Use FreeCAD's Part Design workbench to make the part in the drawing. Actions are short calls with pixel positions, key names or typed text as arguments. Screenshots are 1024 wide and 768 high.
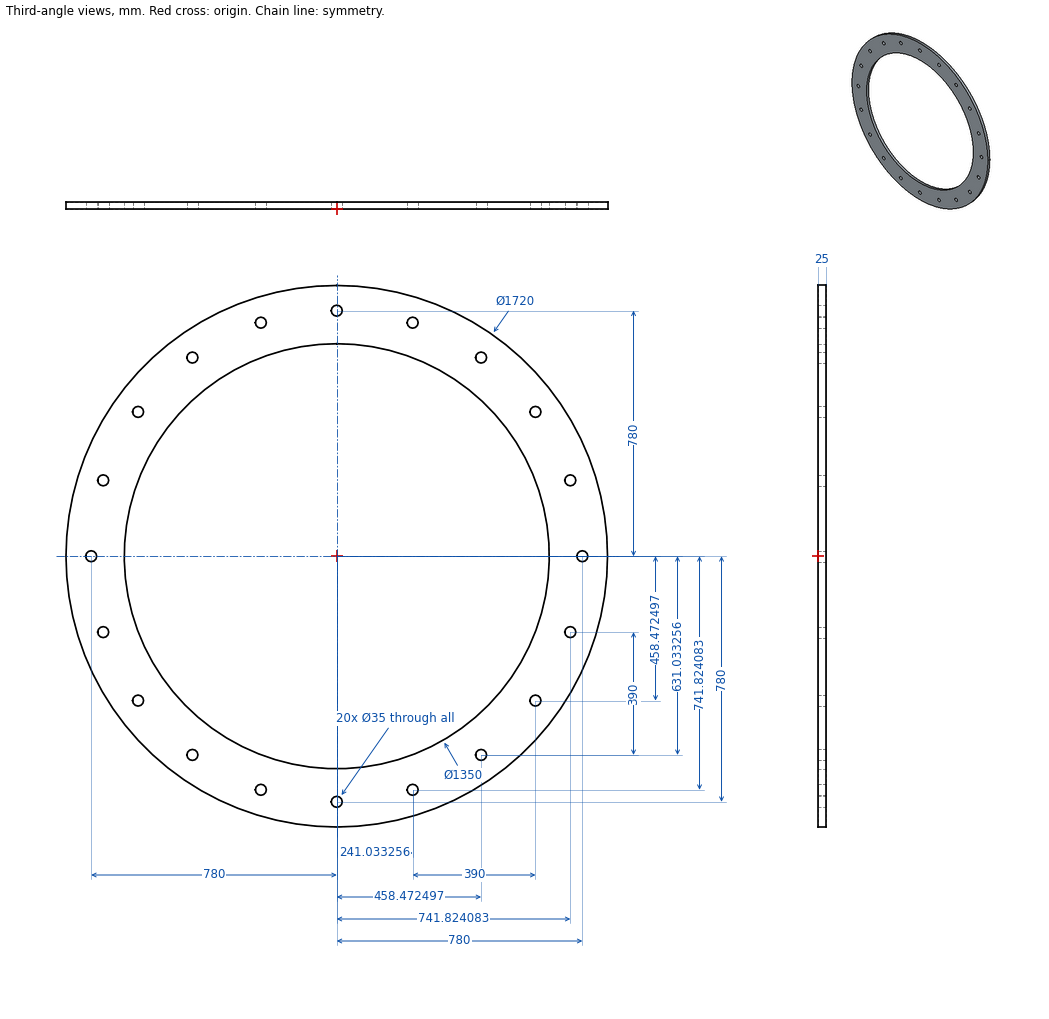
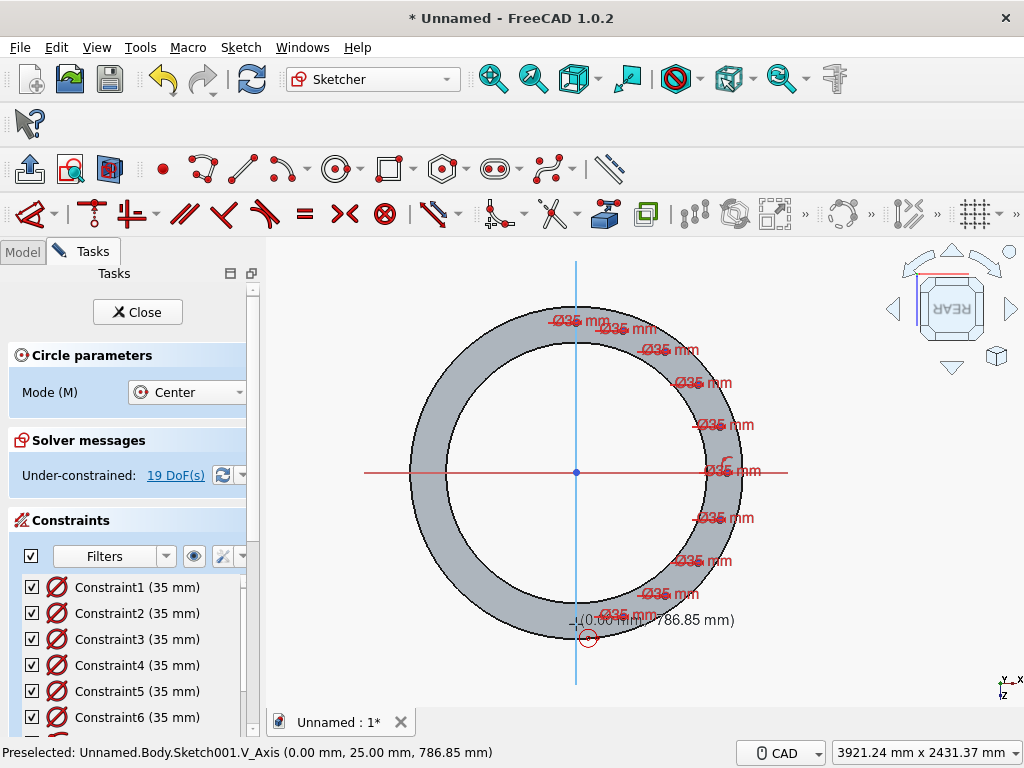
scroll(580, 623, up, 9)
move(576, 616)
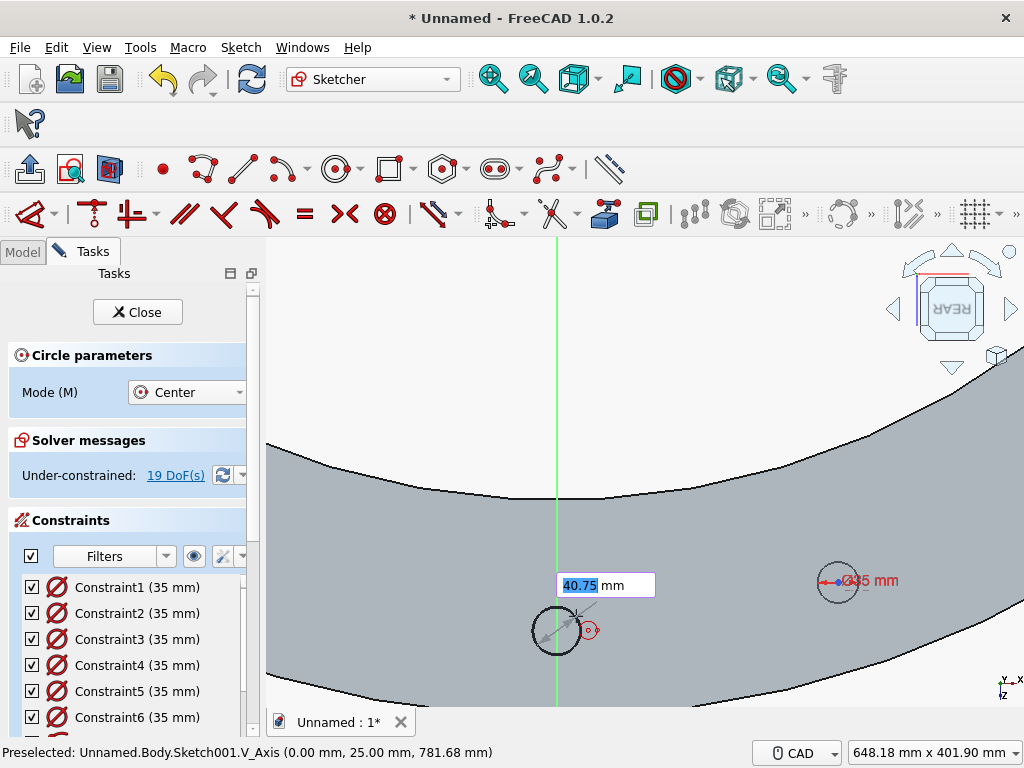
text(35)
key(Return)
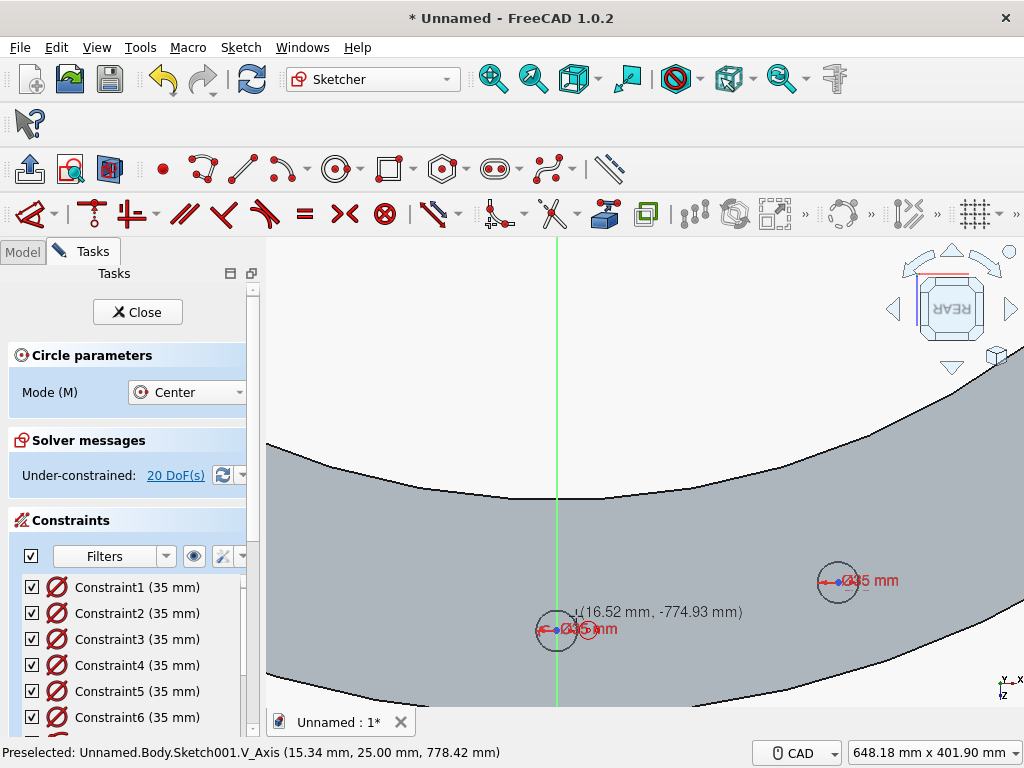
scroll(580, 623, down, 9)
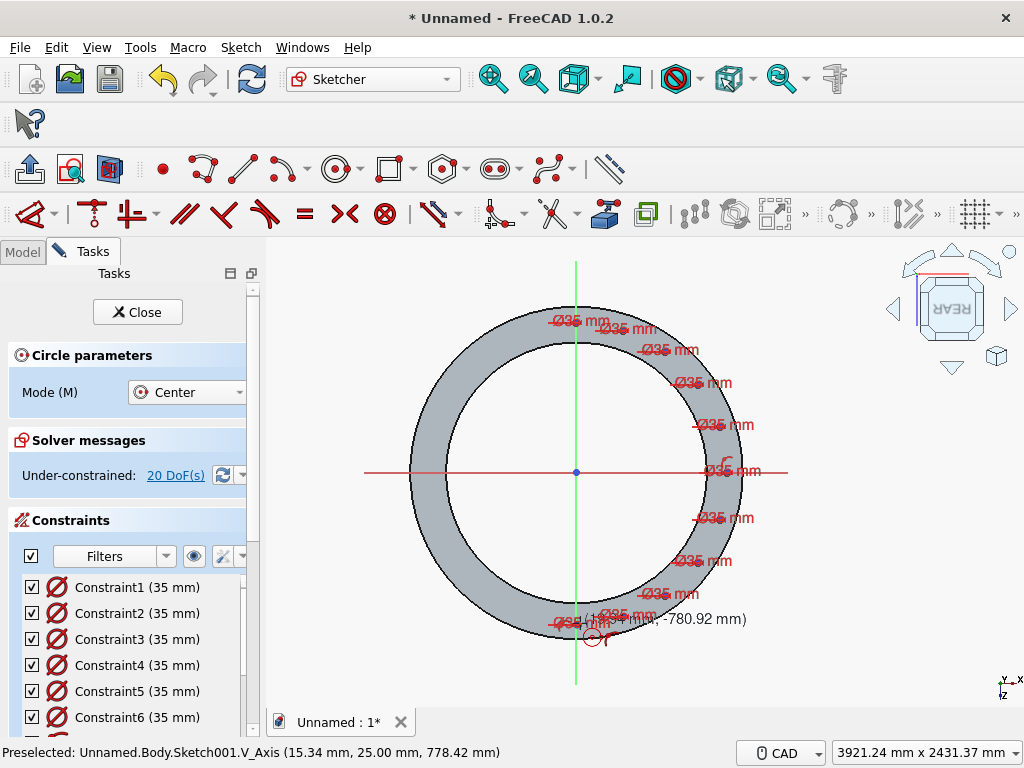
scroll(530, 616, up, 10)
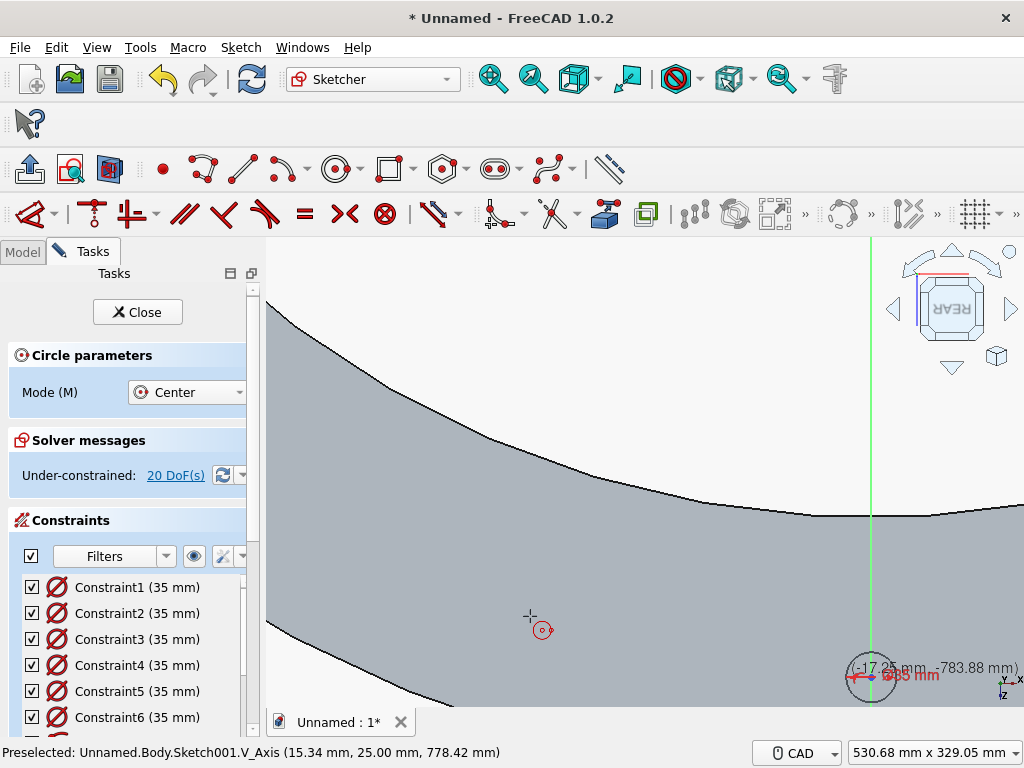
scroll(530, 616, down, 10)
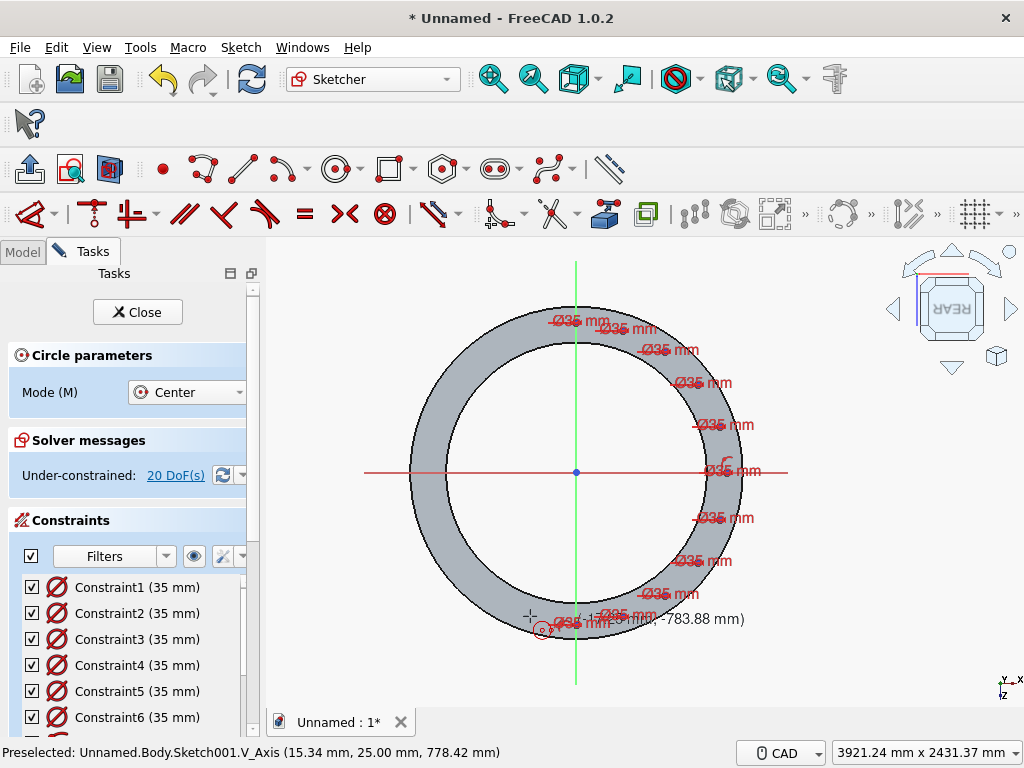
click(530, 616)
move(532, 614)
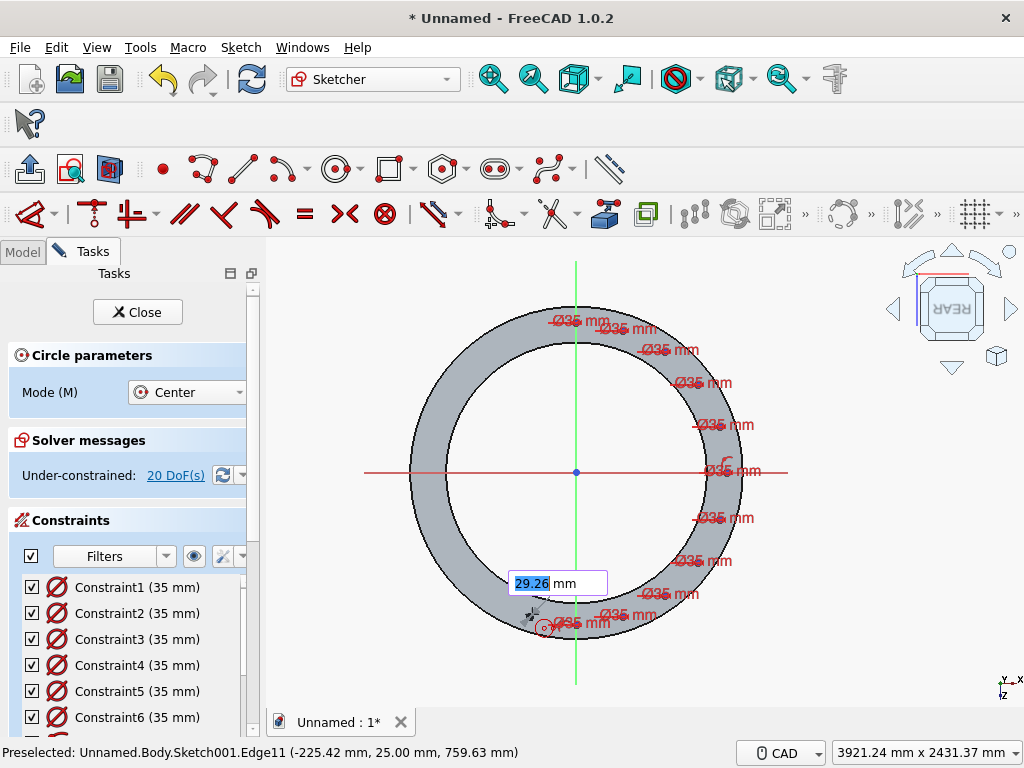
text(35)
key(Return)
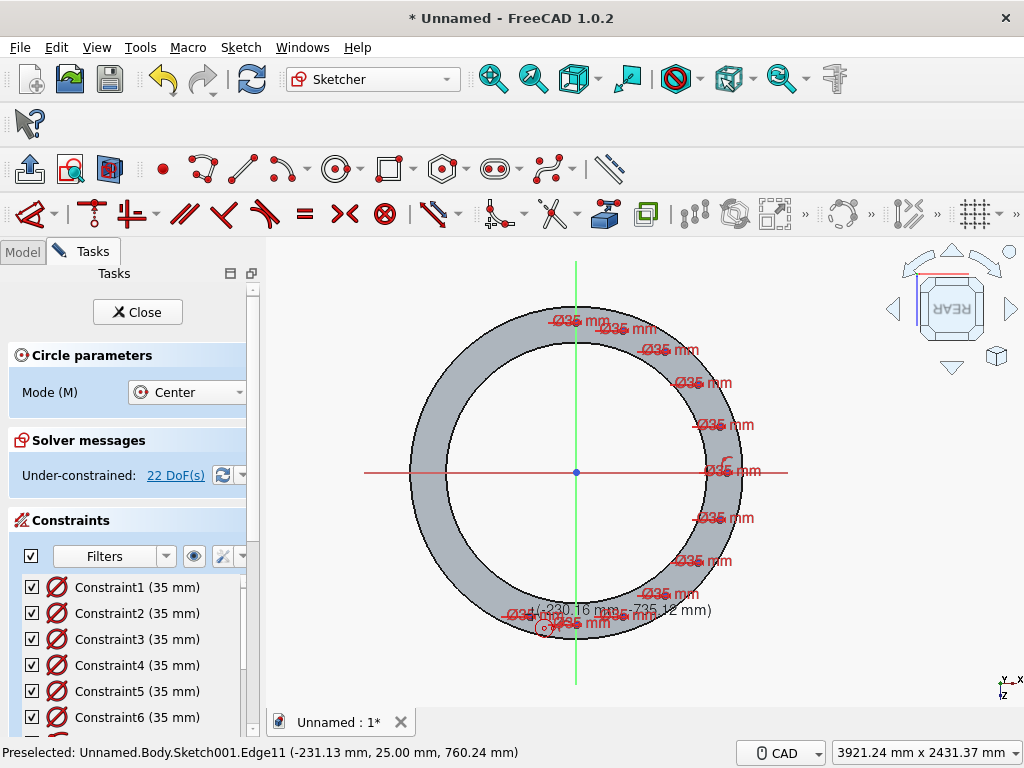
scroll(488, 595, up, 10)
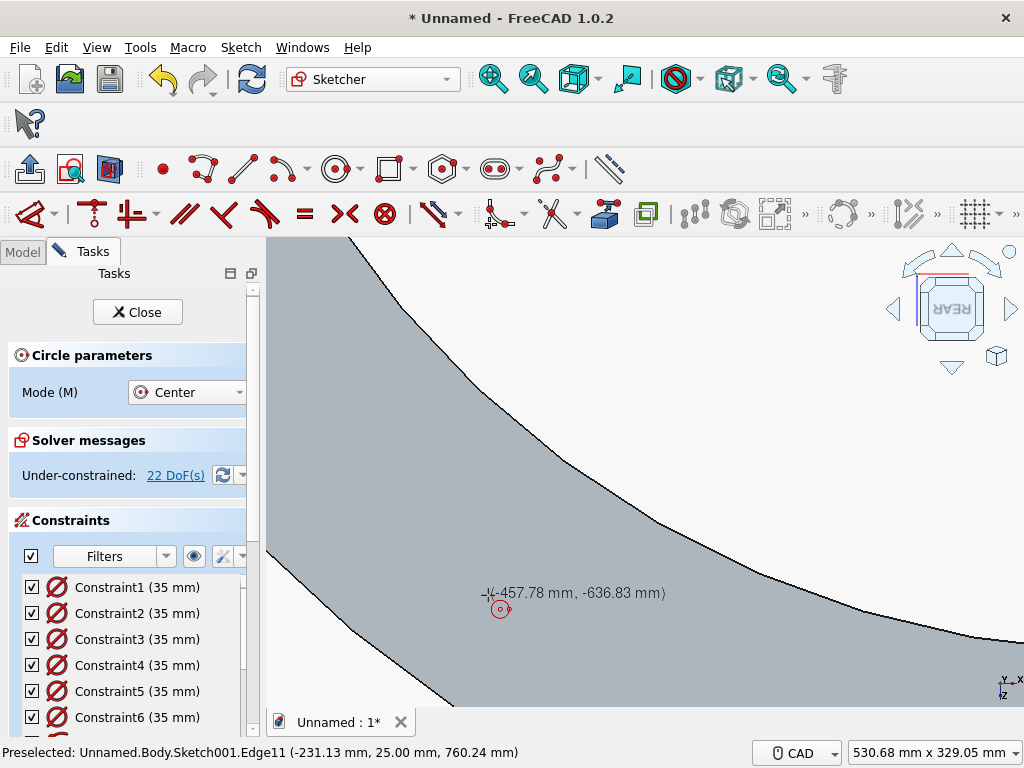
scroll(488, 595, down, 10)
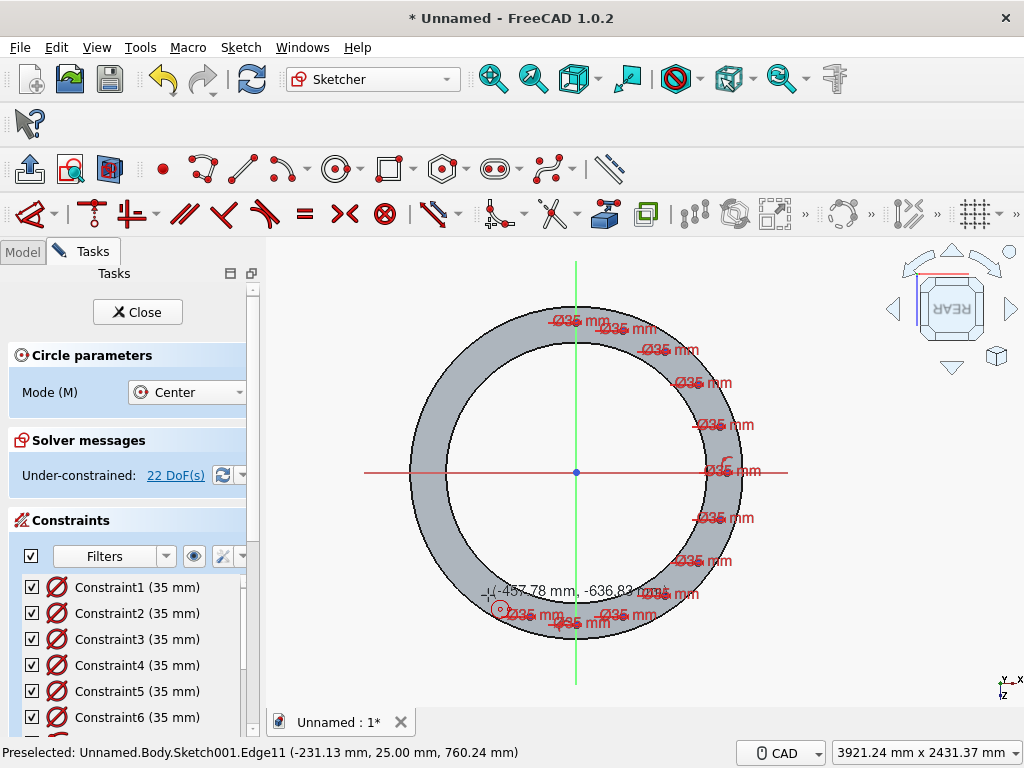
click(488, 595)
move(490, 592)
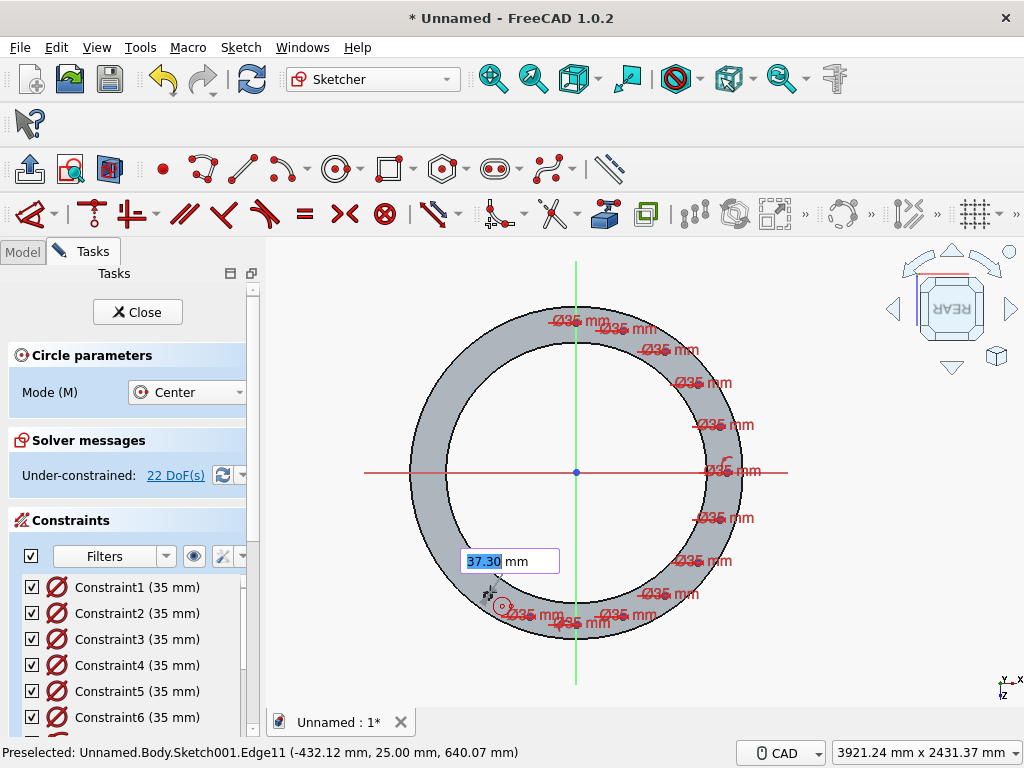
text(35)
key(Return)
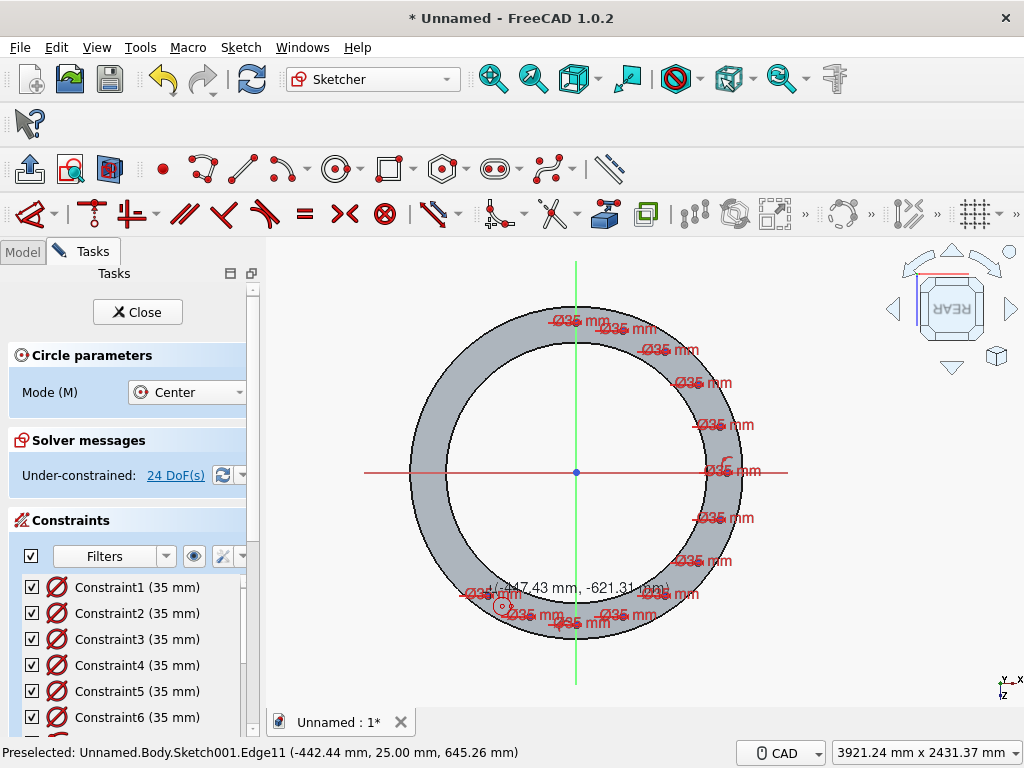
scroll(455, 562, up, 10)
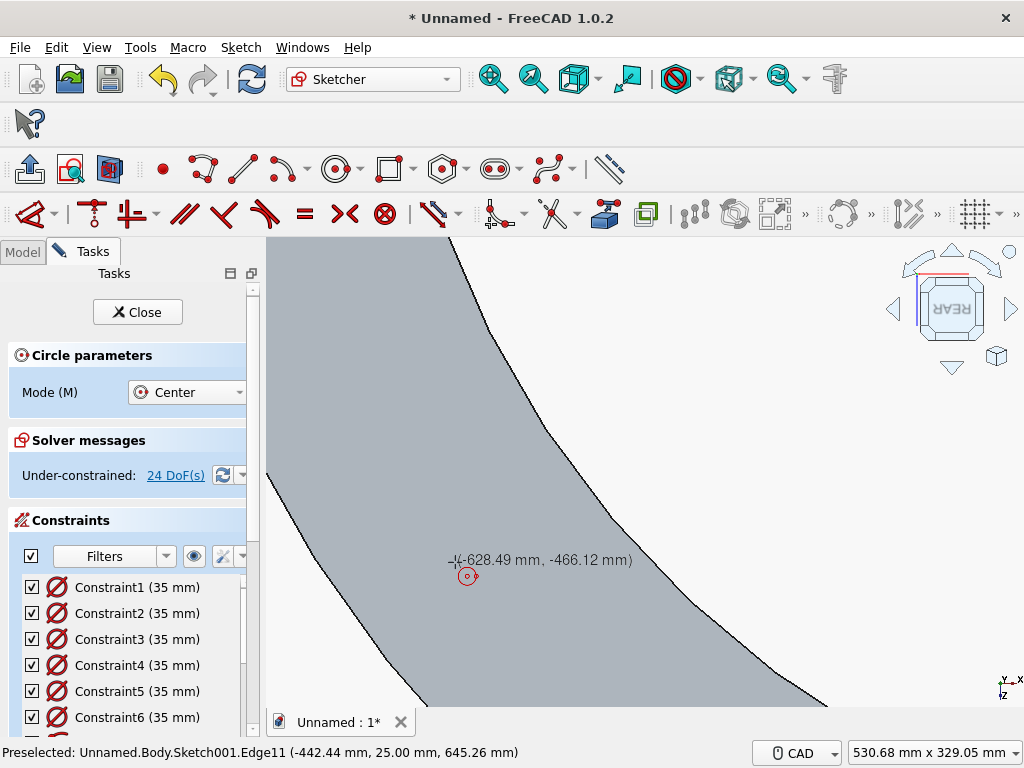
scroll(455, 562, down, 10)